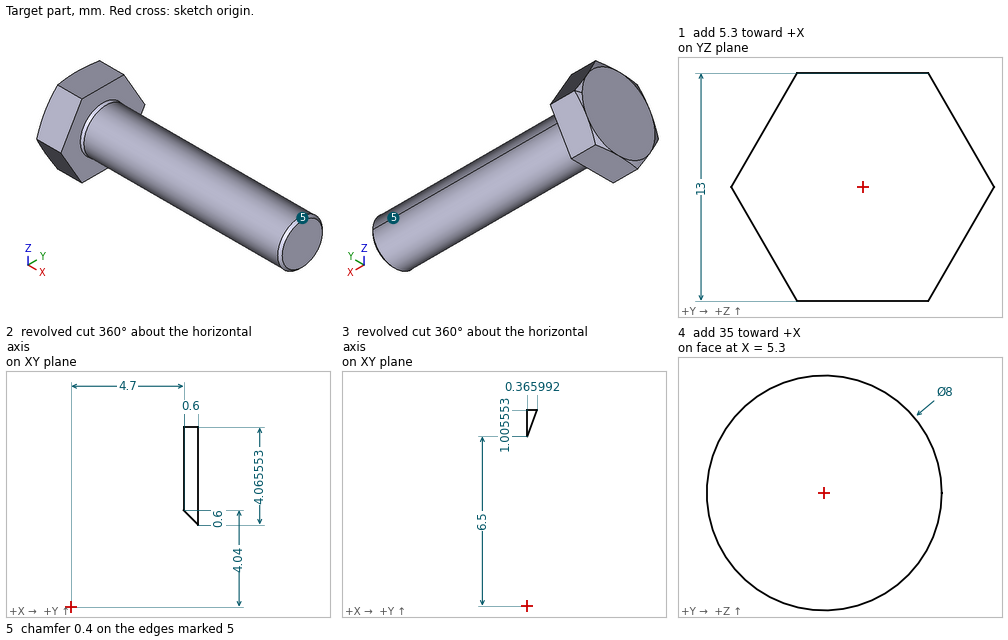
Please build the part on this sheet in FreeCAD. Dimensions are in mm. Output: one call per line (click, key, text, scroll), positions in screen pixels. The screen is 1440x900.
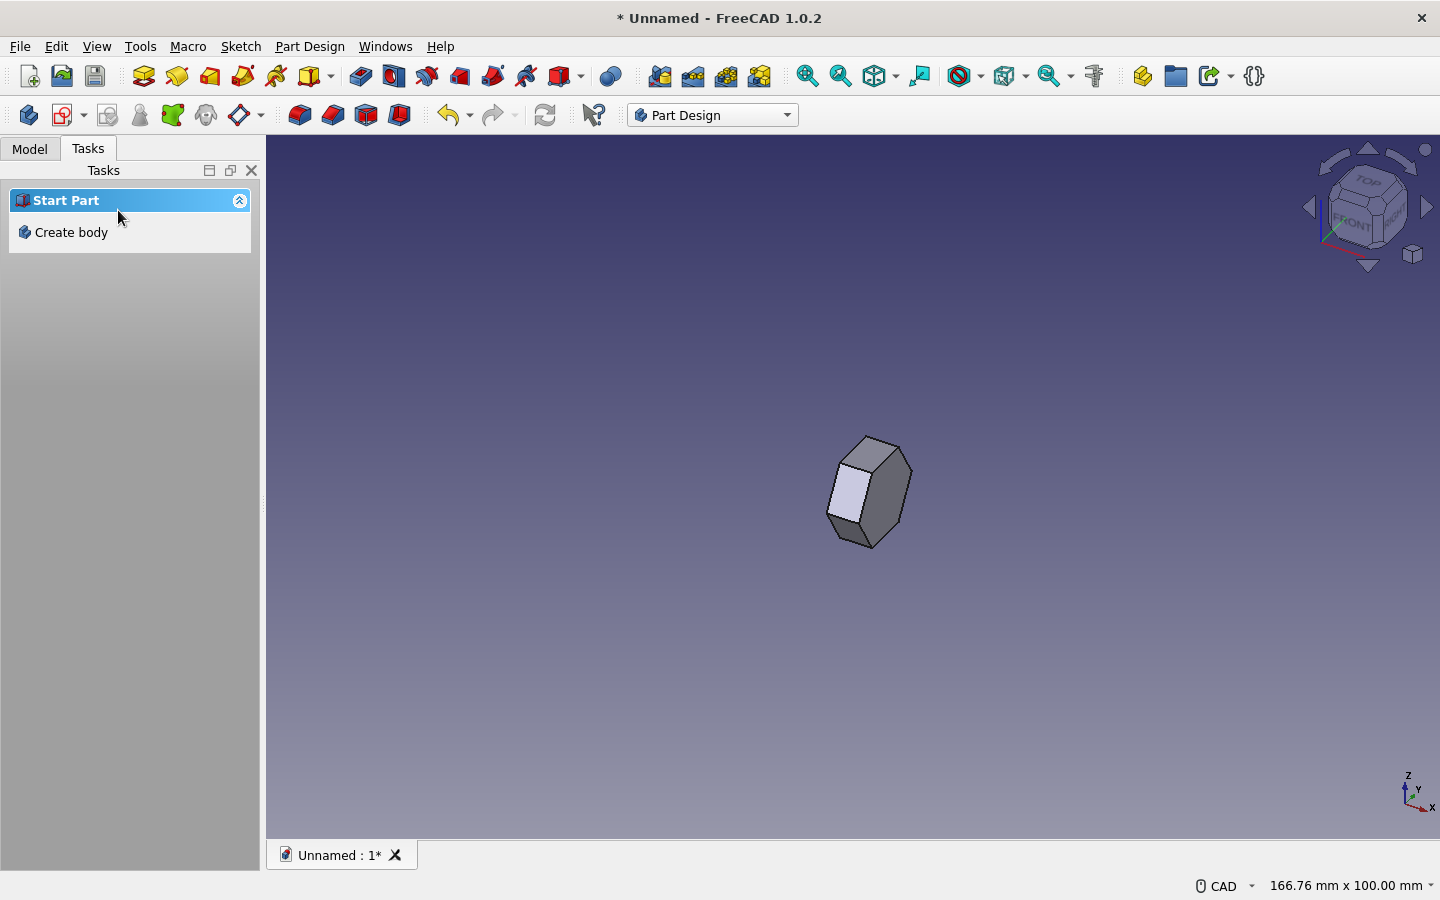
key(v)
key(f)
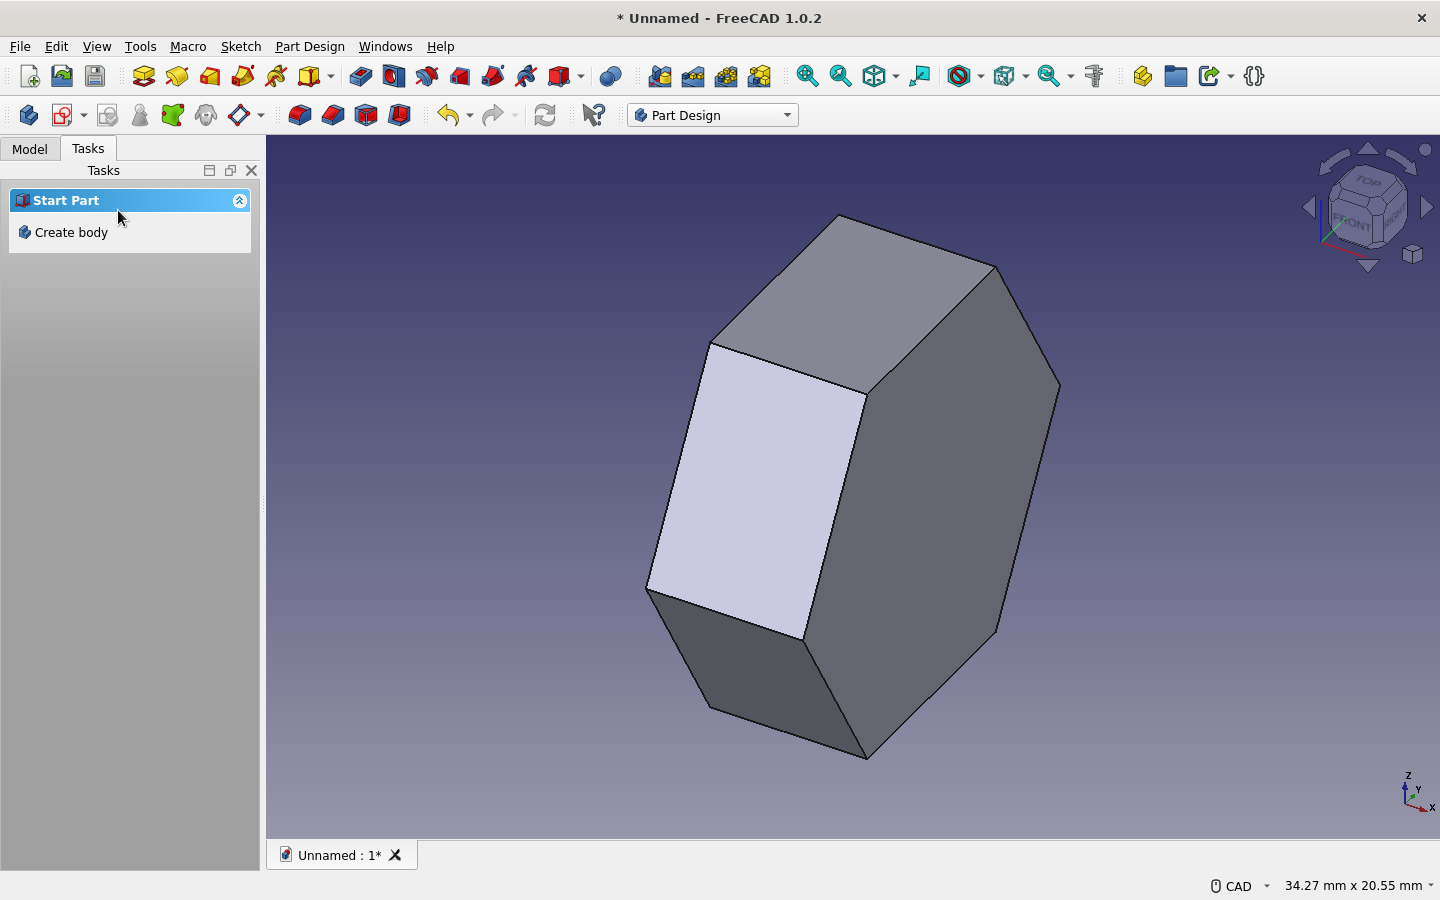
click(62, 116)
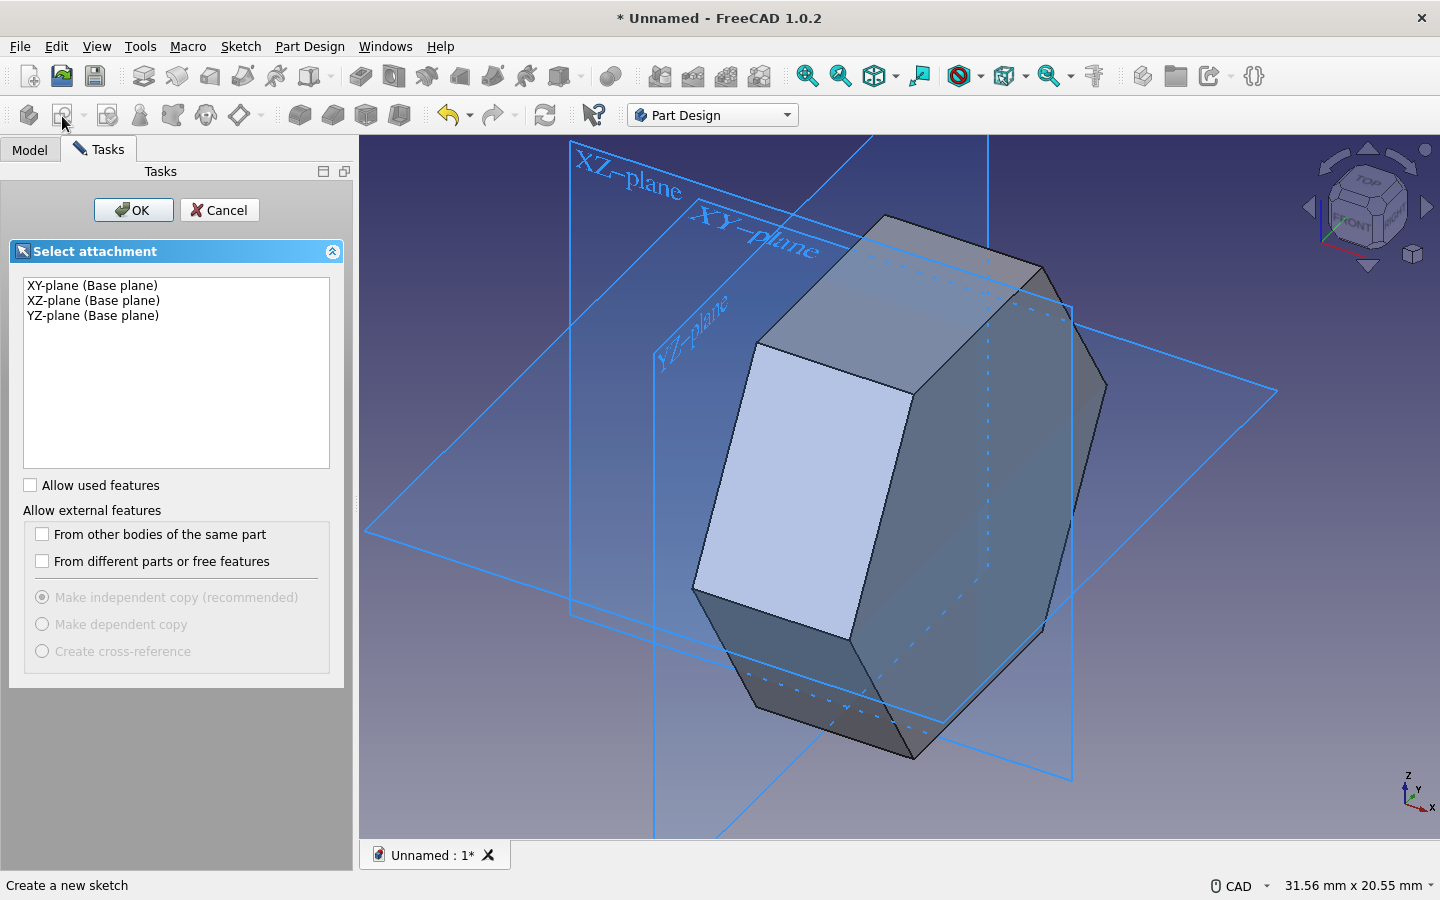
click(84, 286)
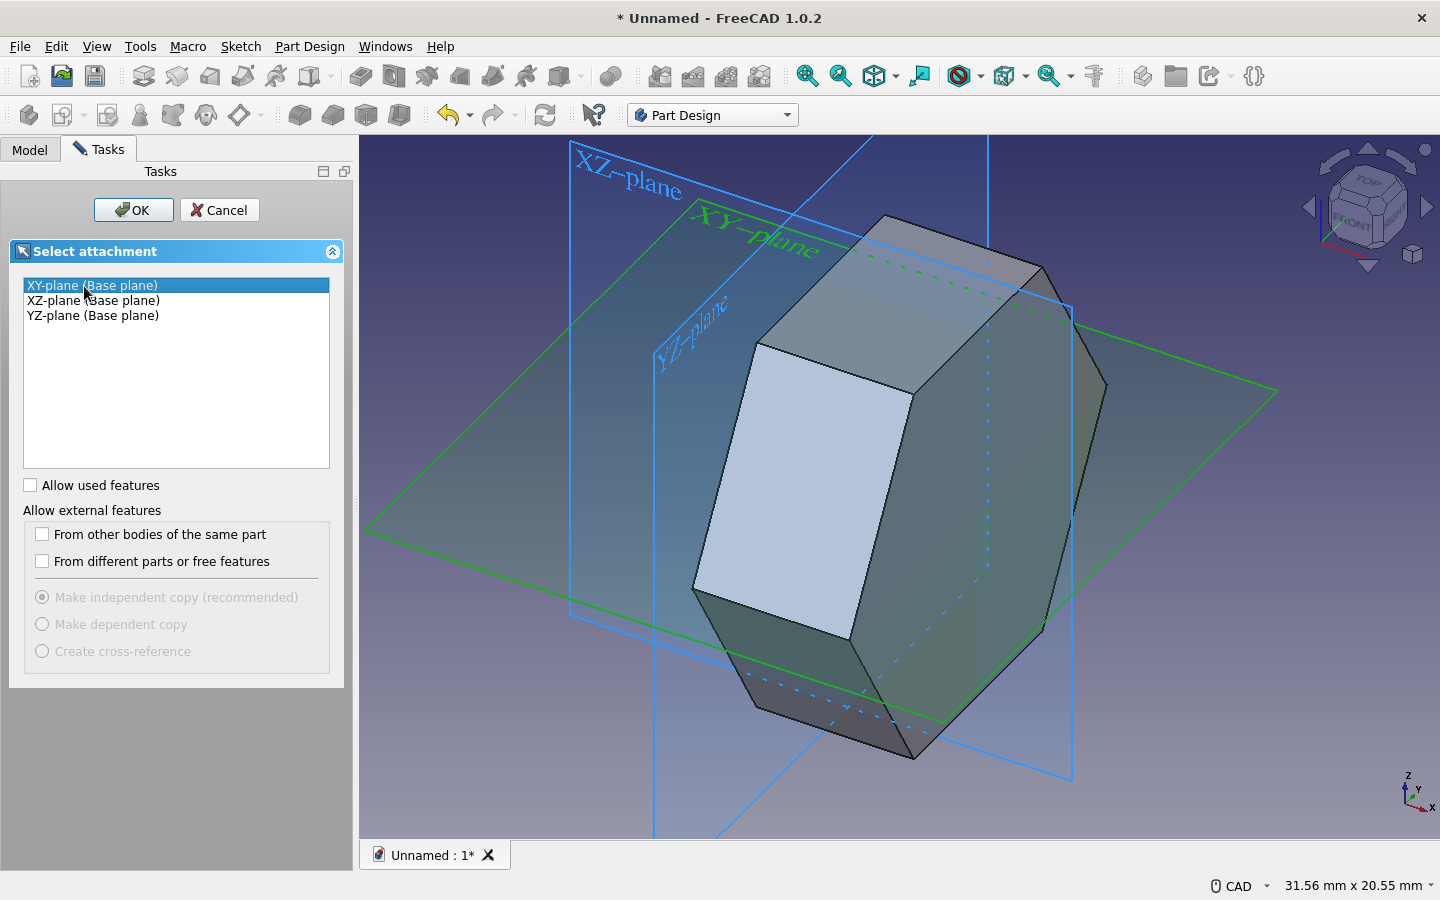
click(134, 210)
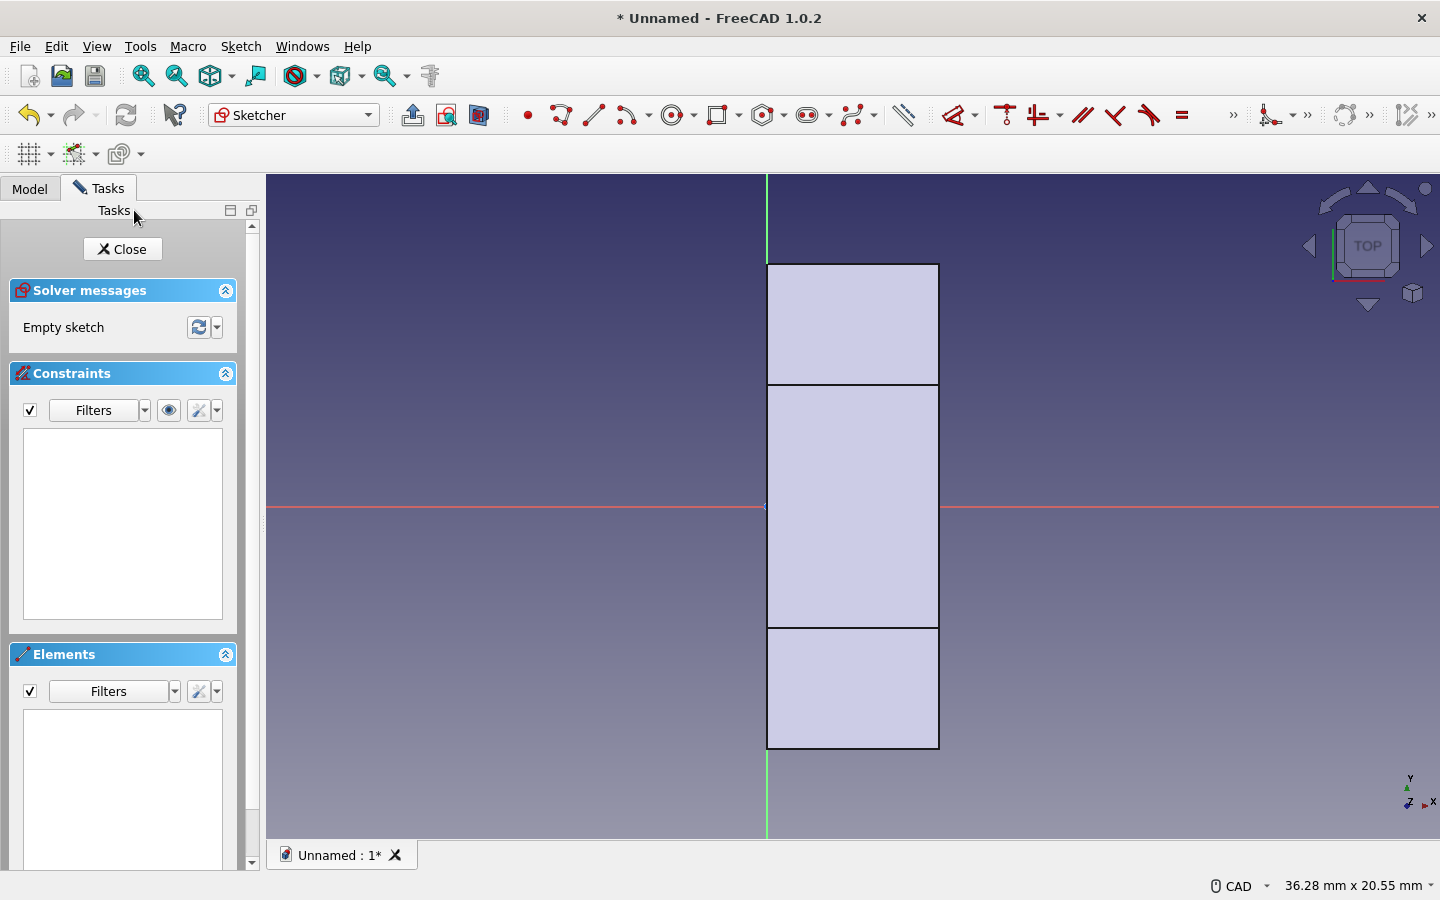
key(q)
key(s)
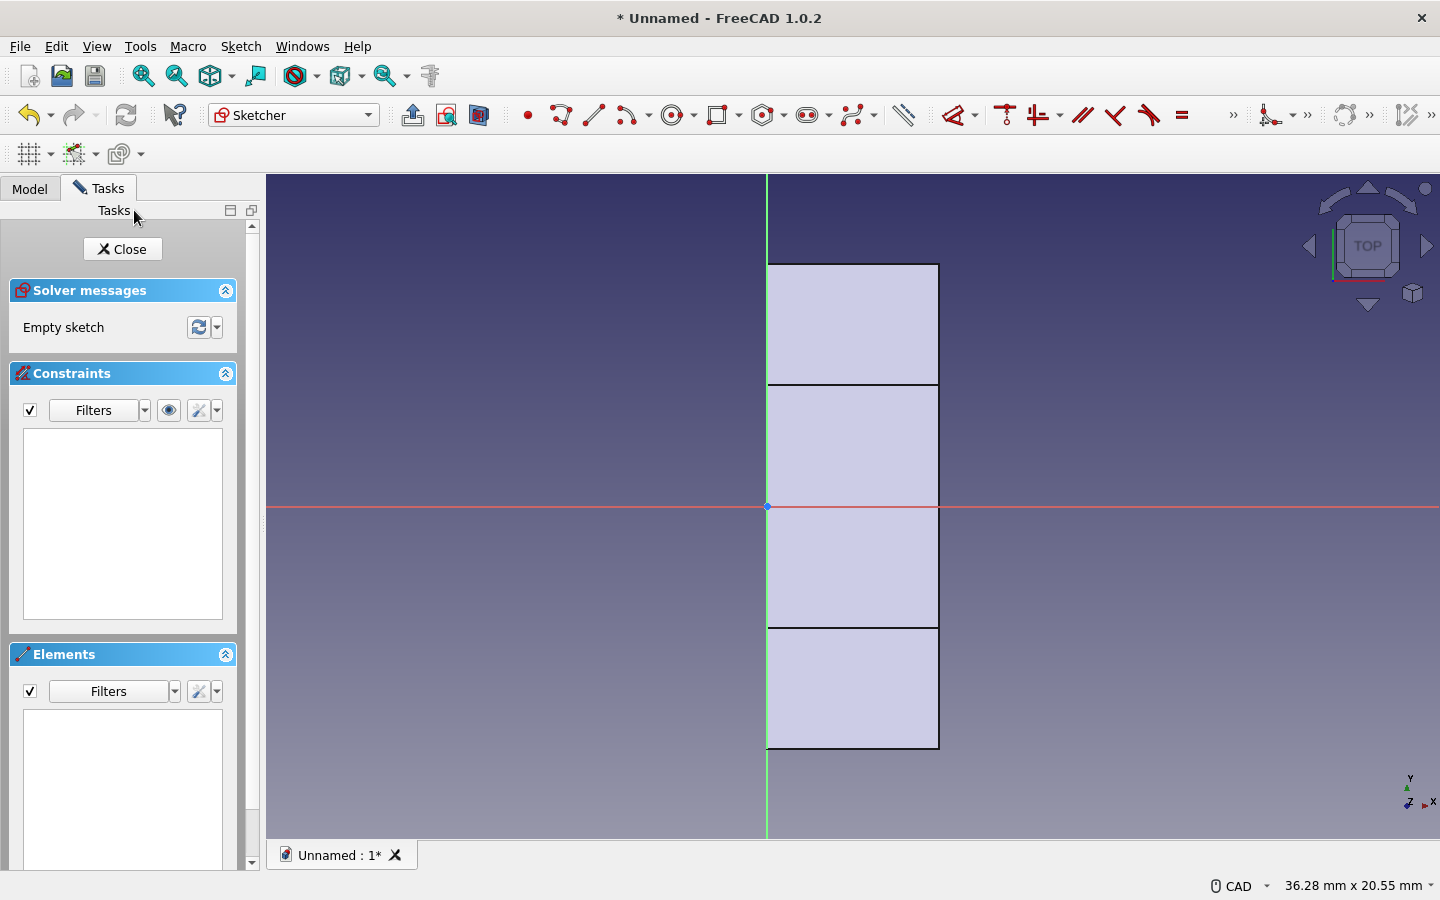
scroll(936, 237, up, 3)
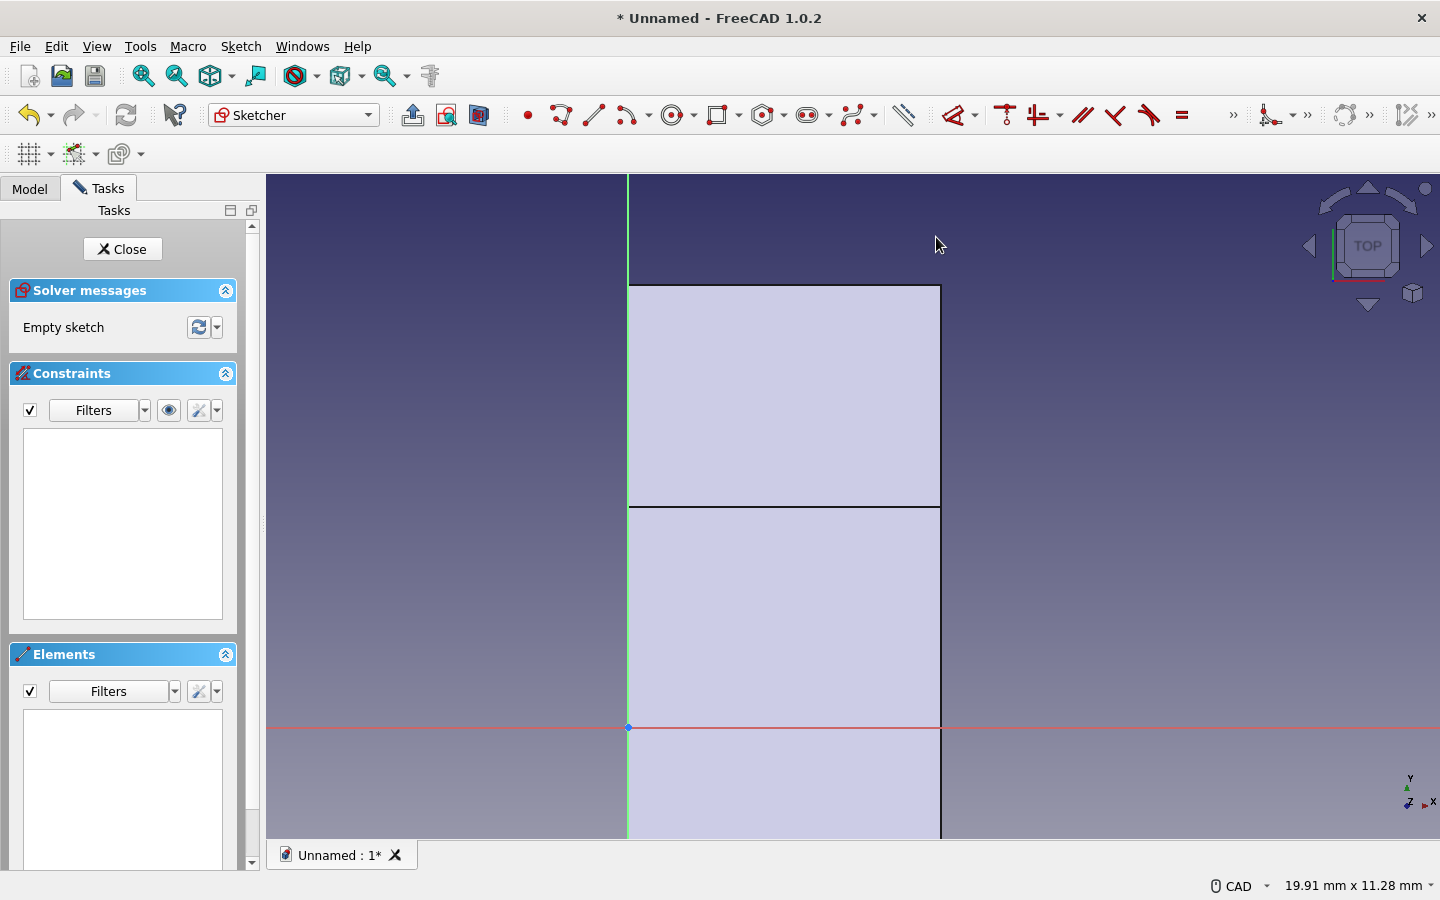
click(561, 116)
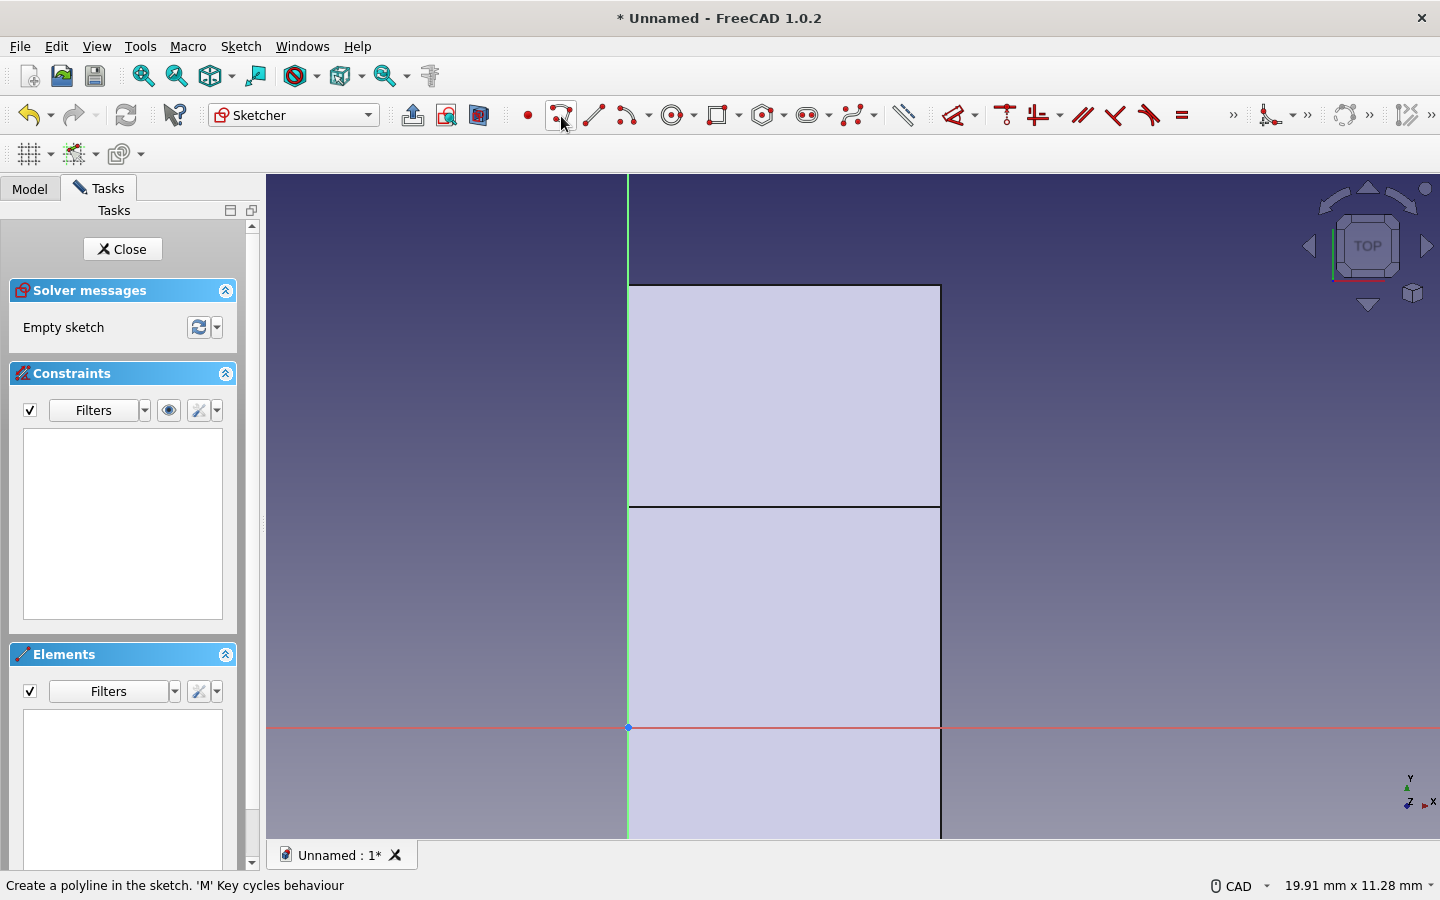
click(905, 490)
click(941, 525)
click(941, 285)
click(905, 285)
click(905, 491)
key(Escape)
key(Escape)